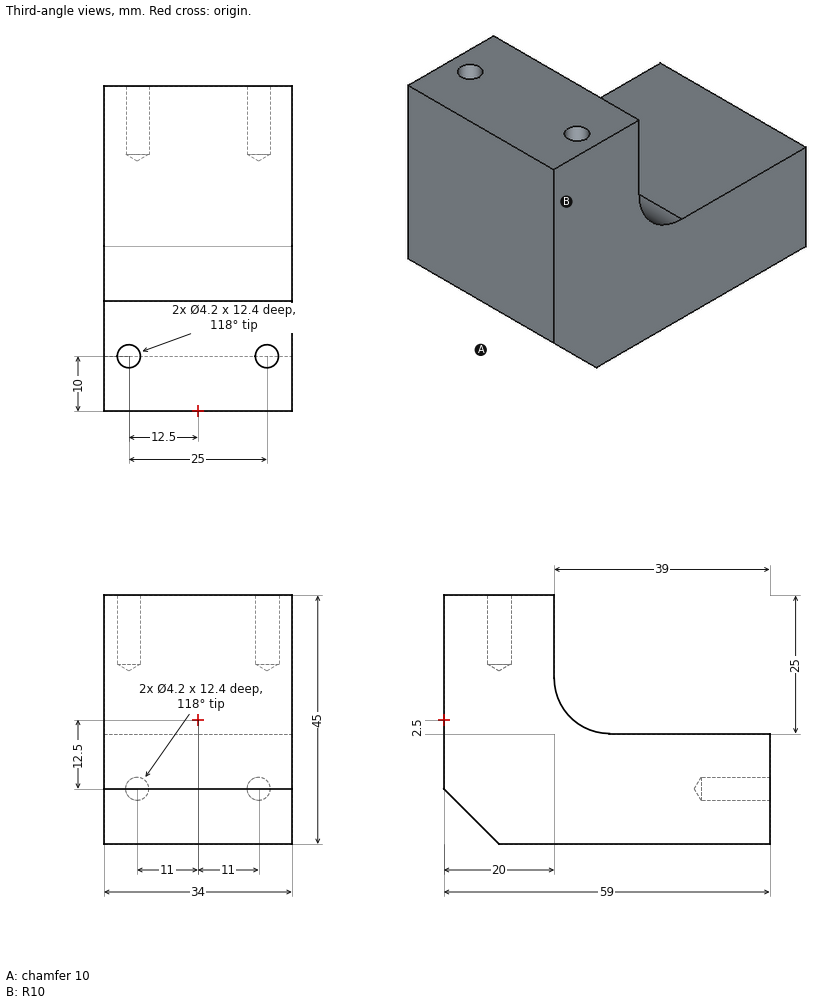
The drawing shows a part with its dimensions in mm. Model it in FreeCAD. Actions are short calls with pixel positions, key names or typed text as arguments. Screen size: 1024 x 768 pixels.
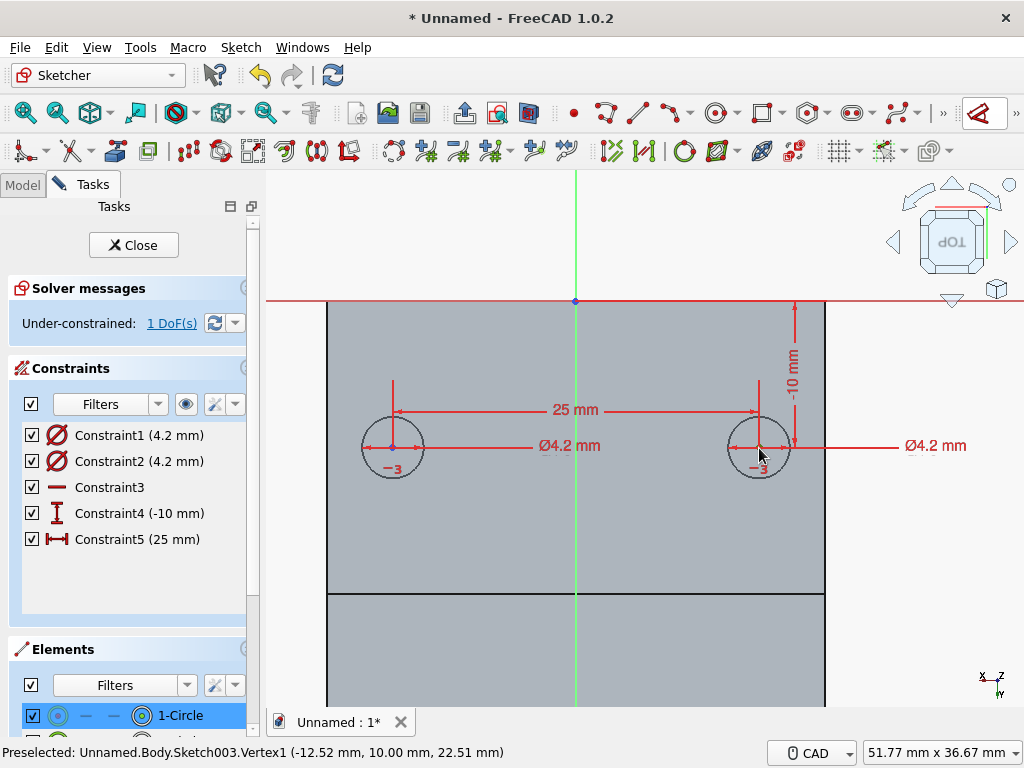
click(1002, 114)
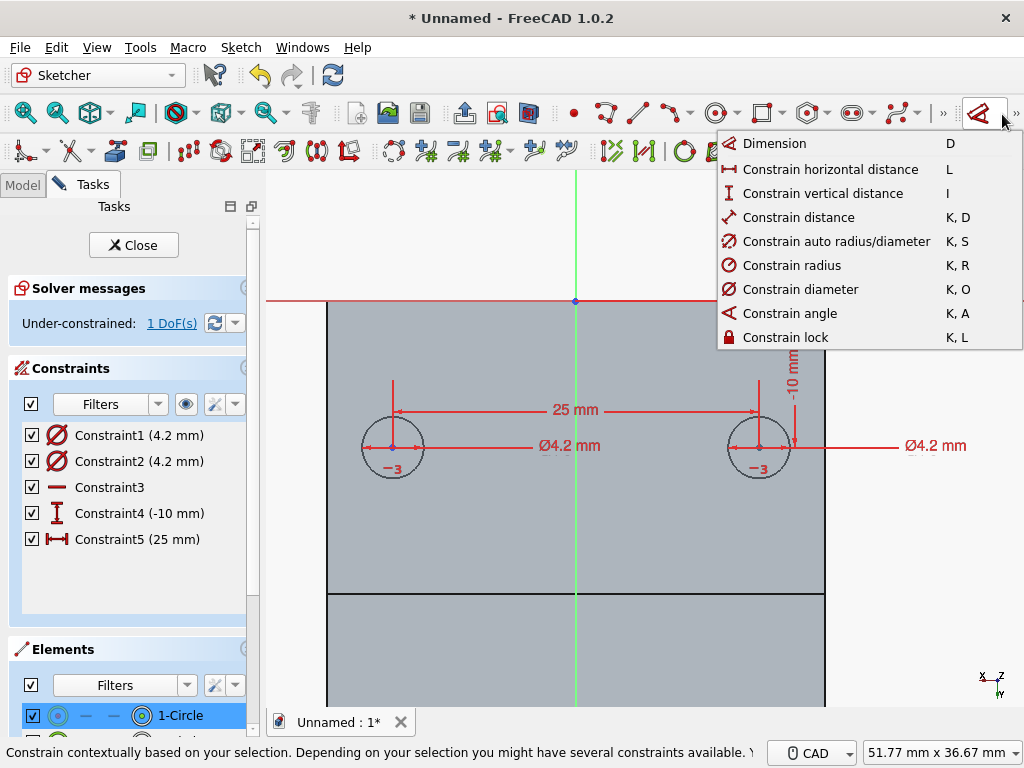
click(870, 169)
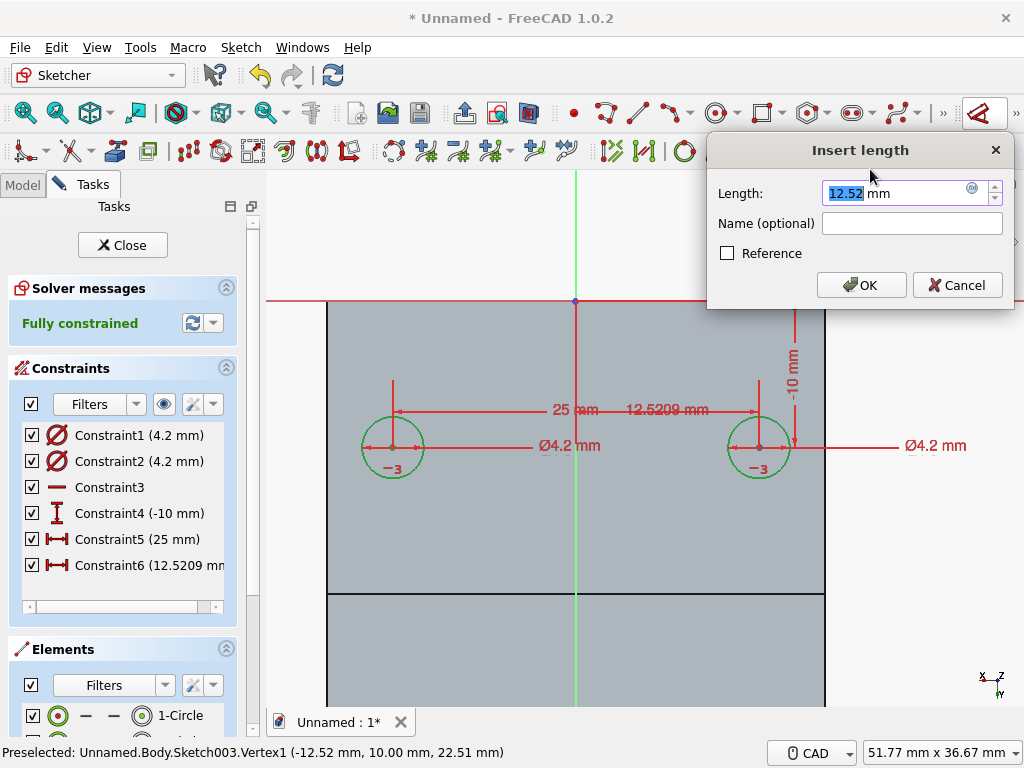
text(12.5)
key(Return)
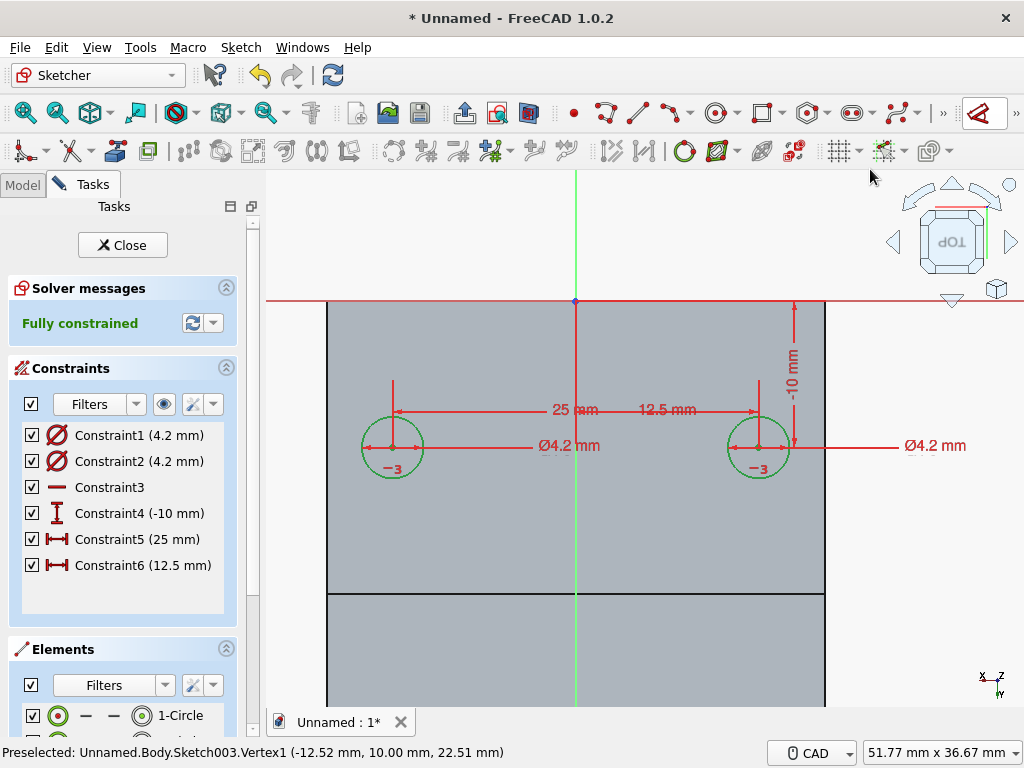
click(123, 245)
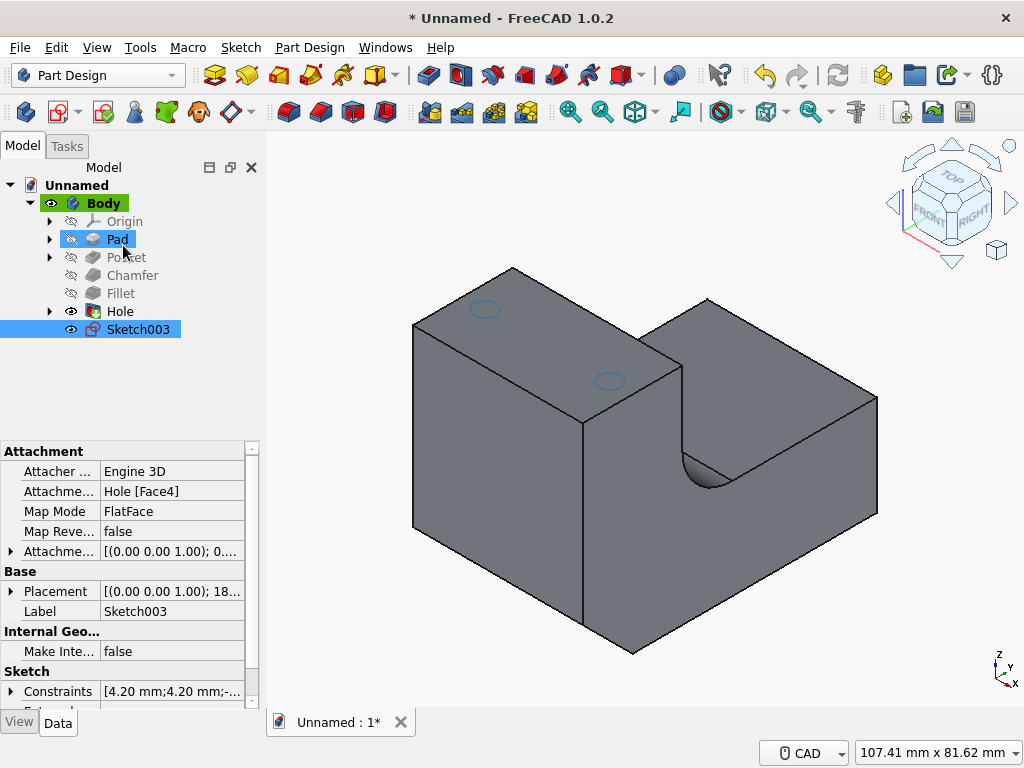
click(462, 76)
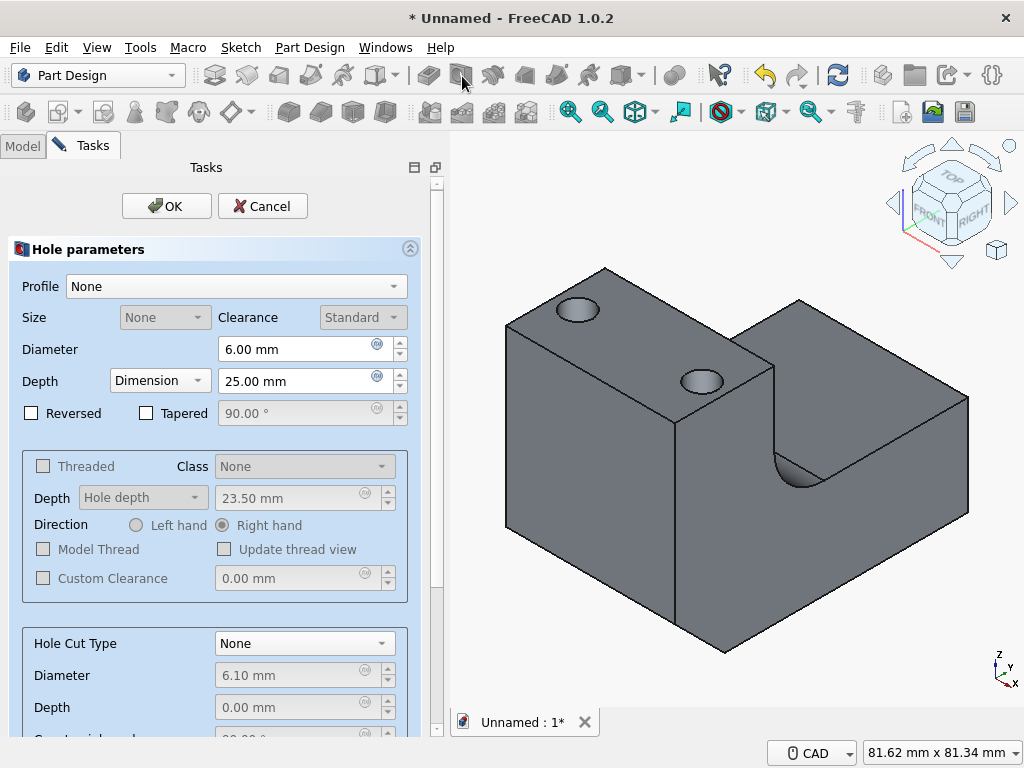
triple_click(305, 349)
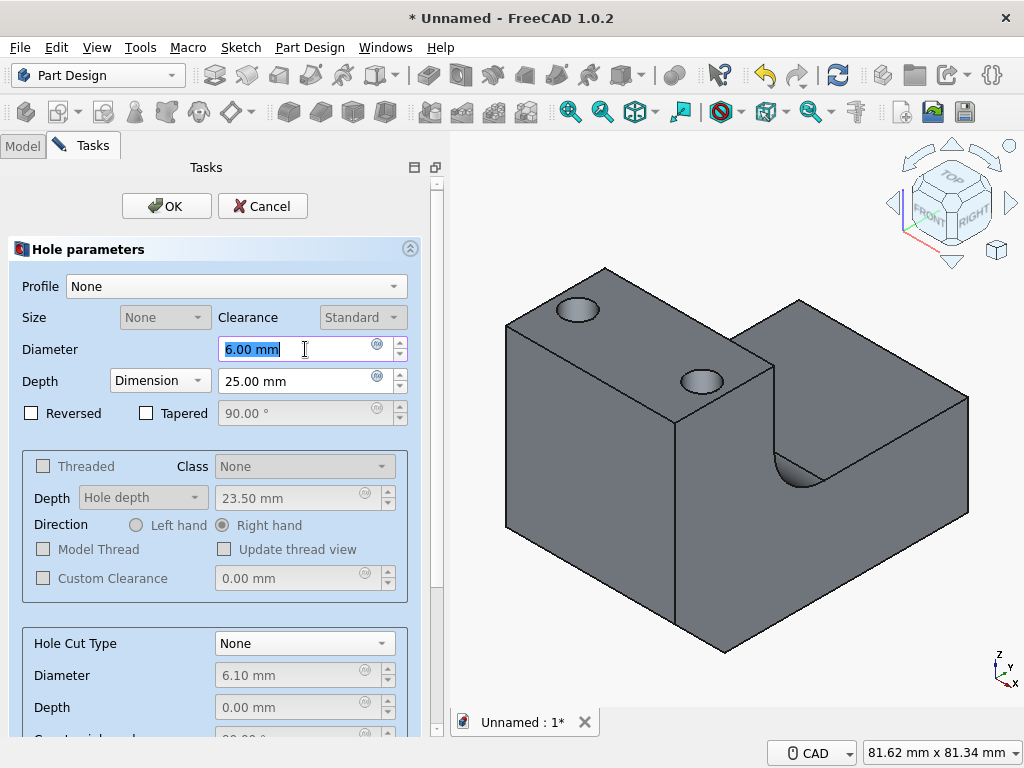
text(4.2)
key(Tab)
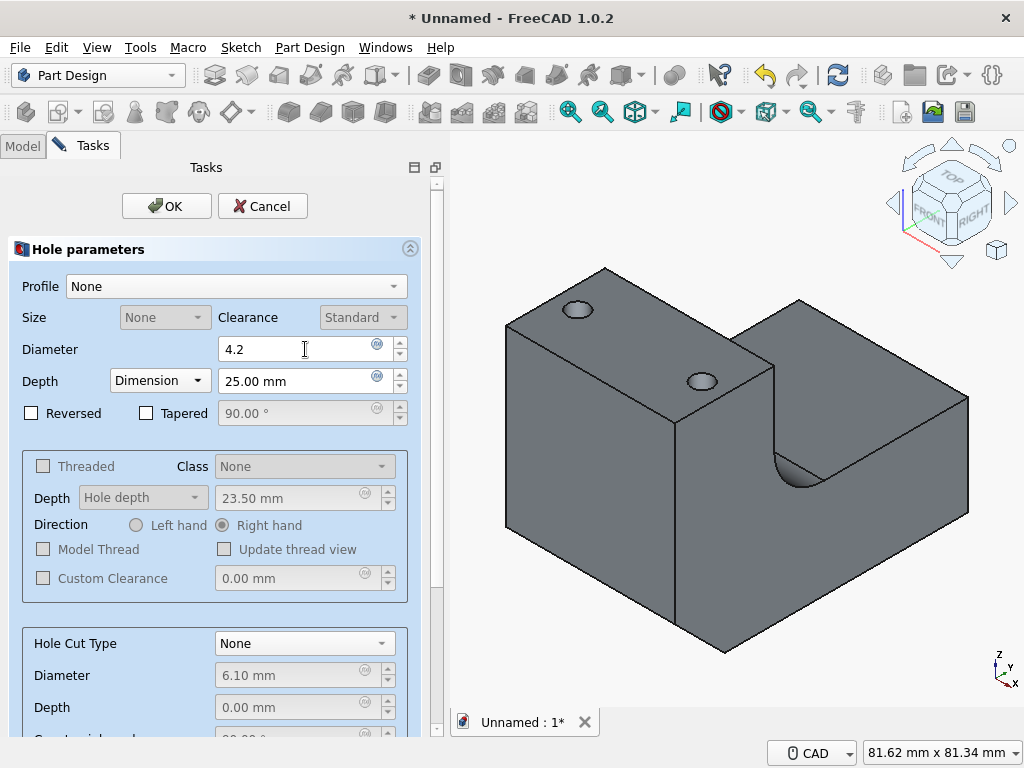
triple_click(305, 381)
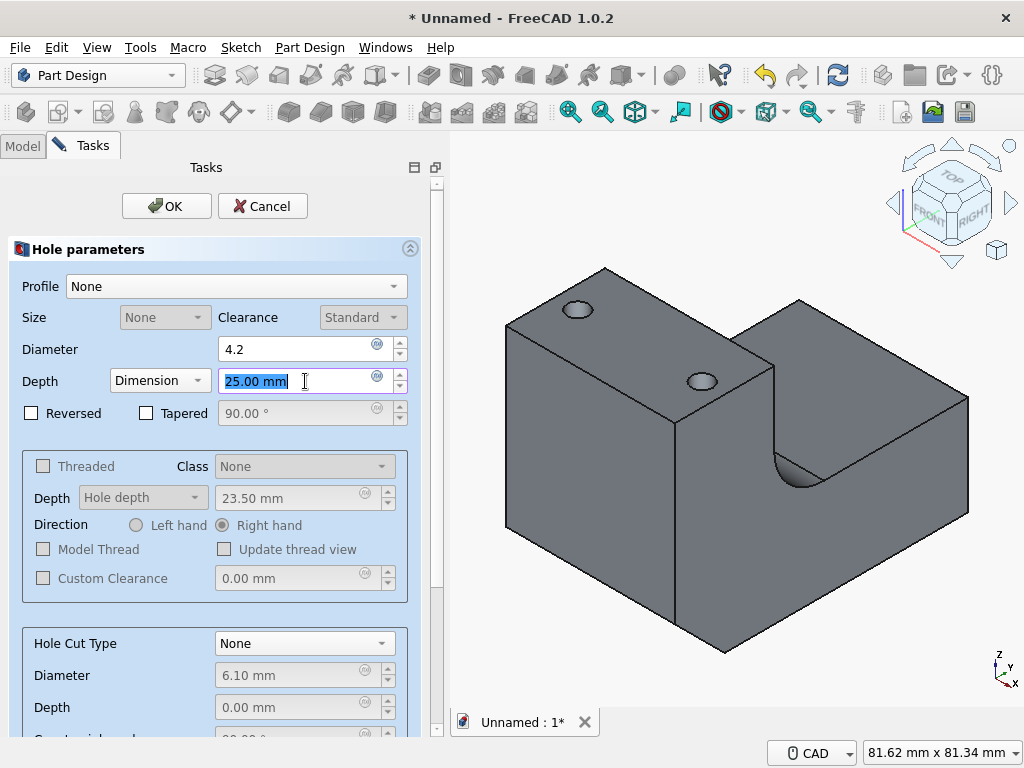
text(12.4)
key(Tab)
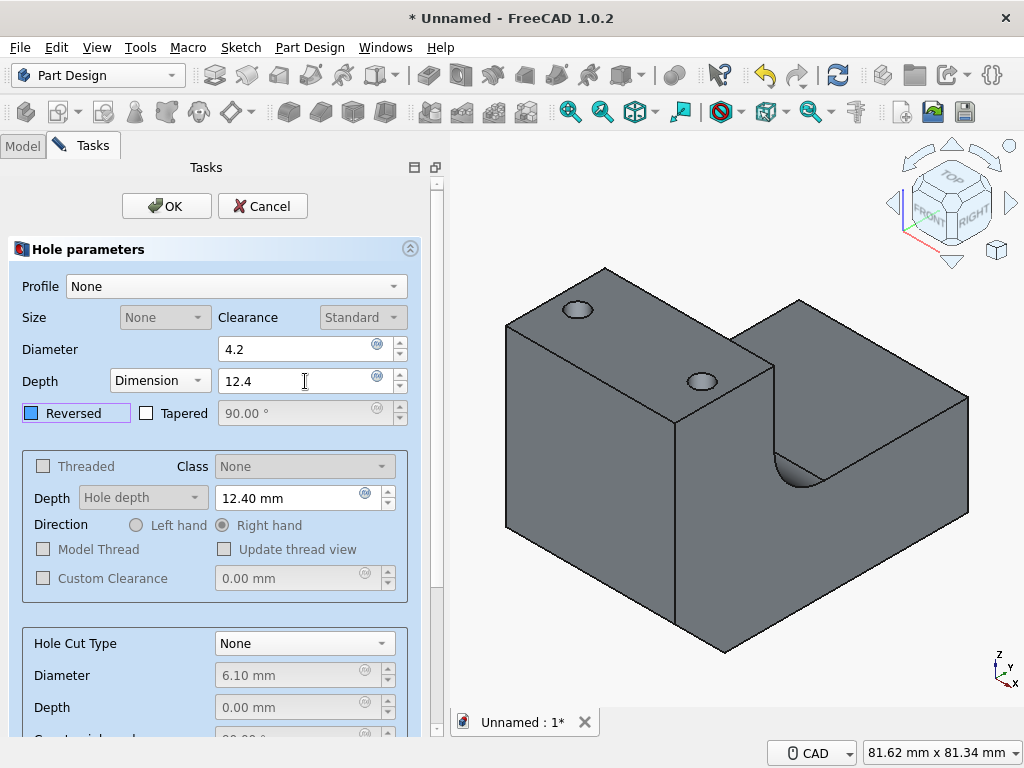
click(167, 206)